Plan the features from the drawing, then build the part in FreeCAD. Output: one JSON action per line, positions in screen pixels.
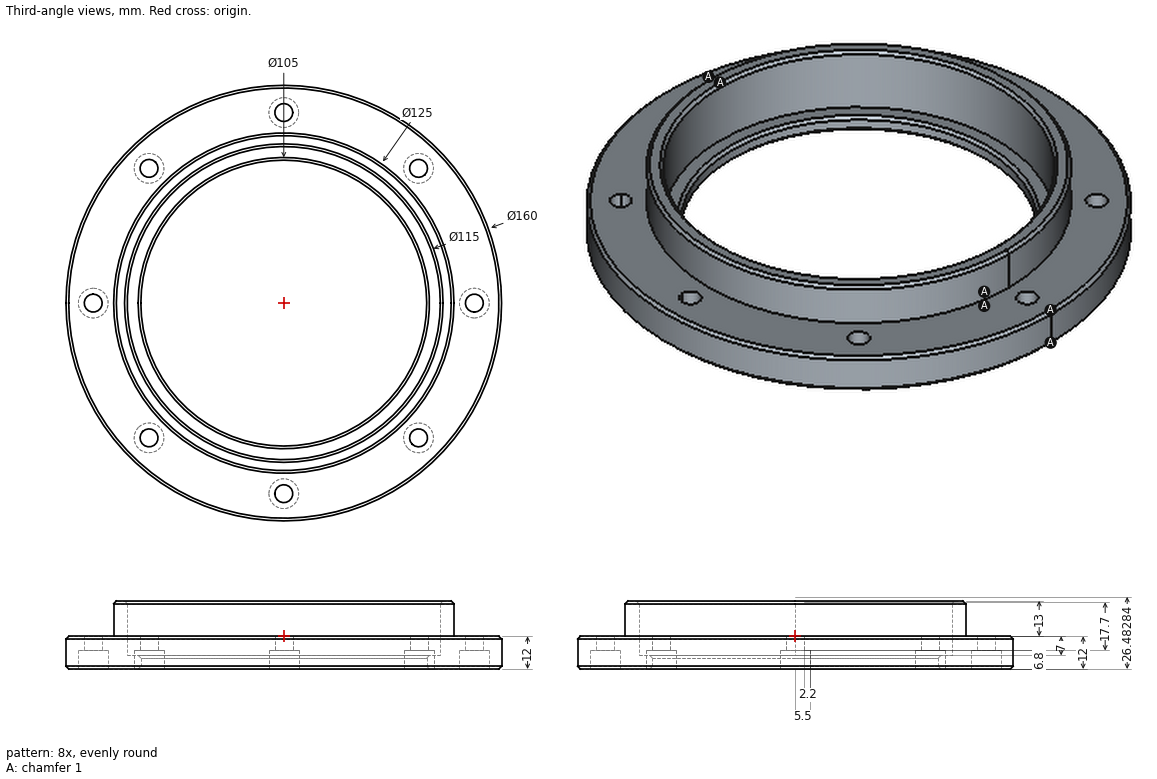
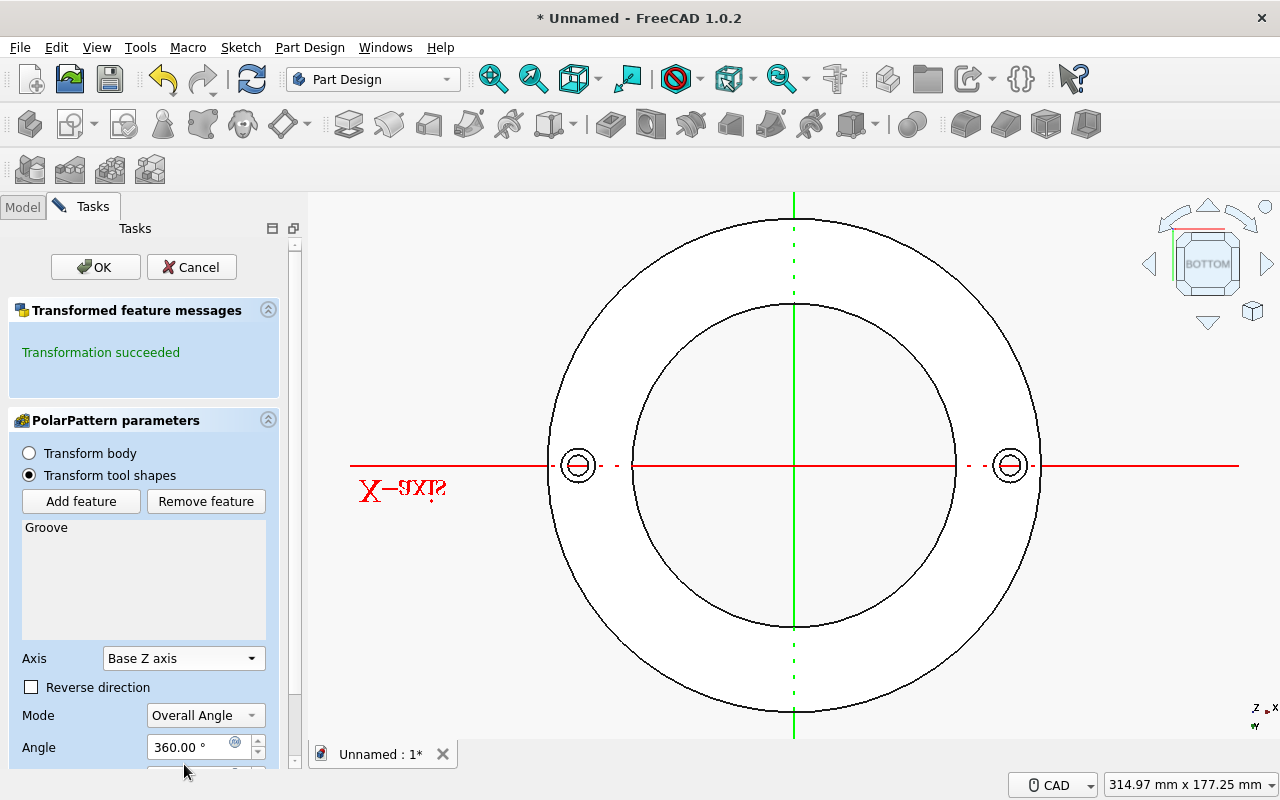
{"action": "scroll", "coordinate": [295, 503], "scroll_direction": "down", "scroll_amount": 2}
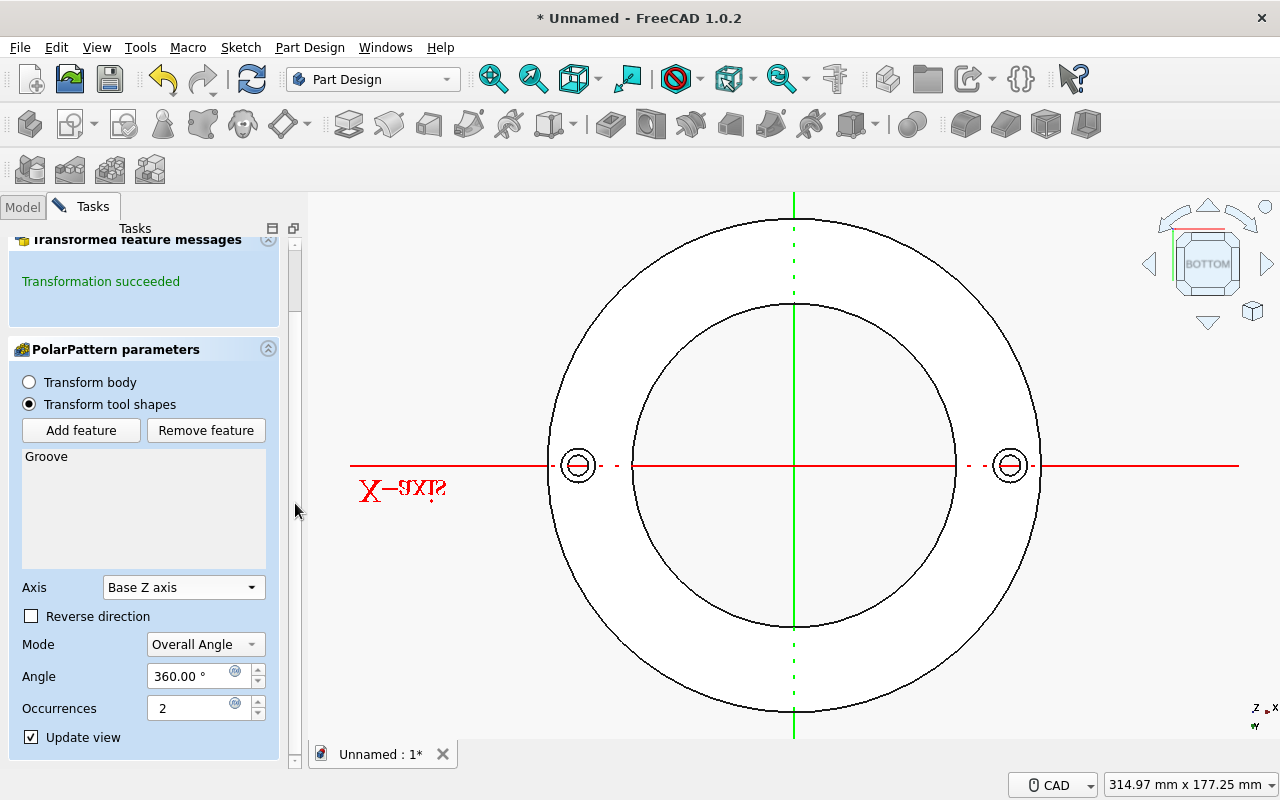
{"action": "triple_click", "coordinate": [198, 708]}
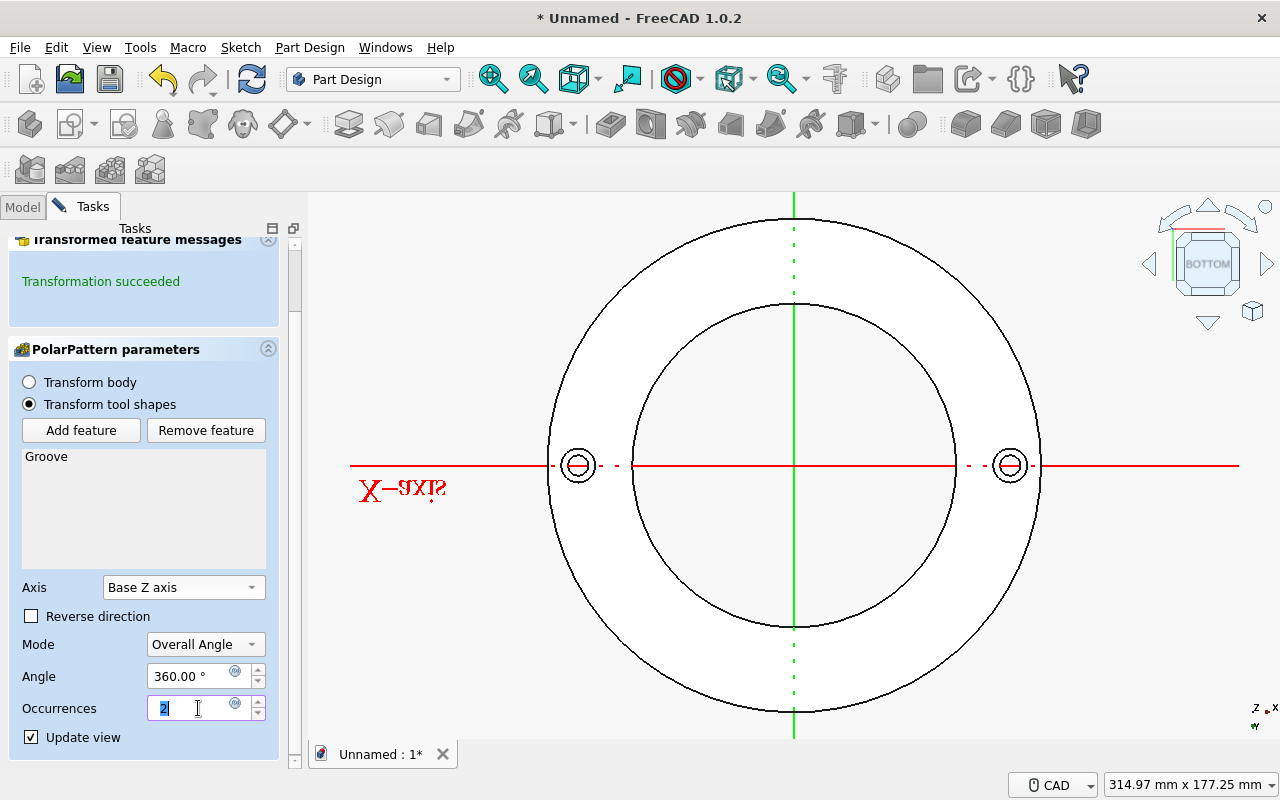
{"action": "type", "text": "8"}
{"action": "key", "text": "Tab"}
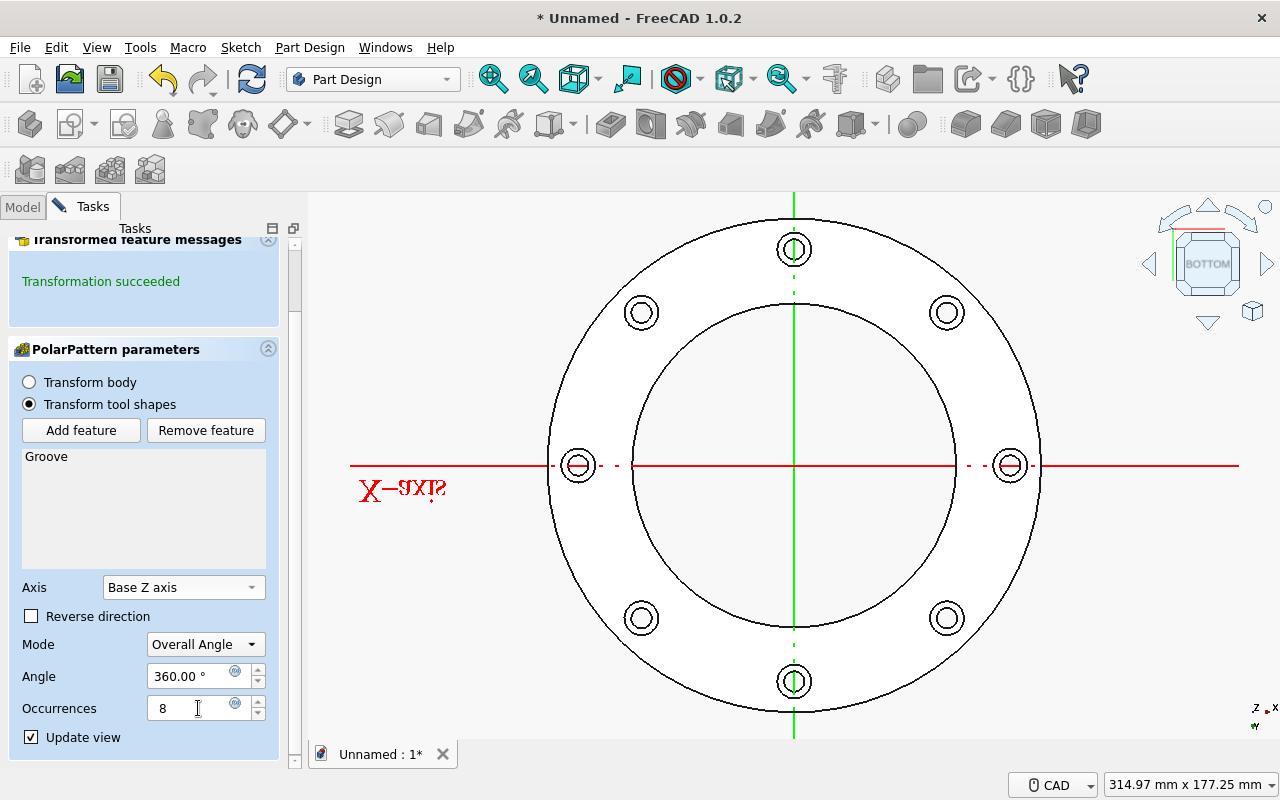
{"action": "scroll", "coordinate": [295, 503], "scroll_direction": "up", "scroll_amount": 2}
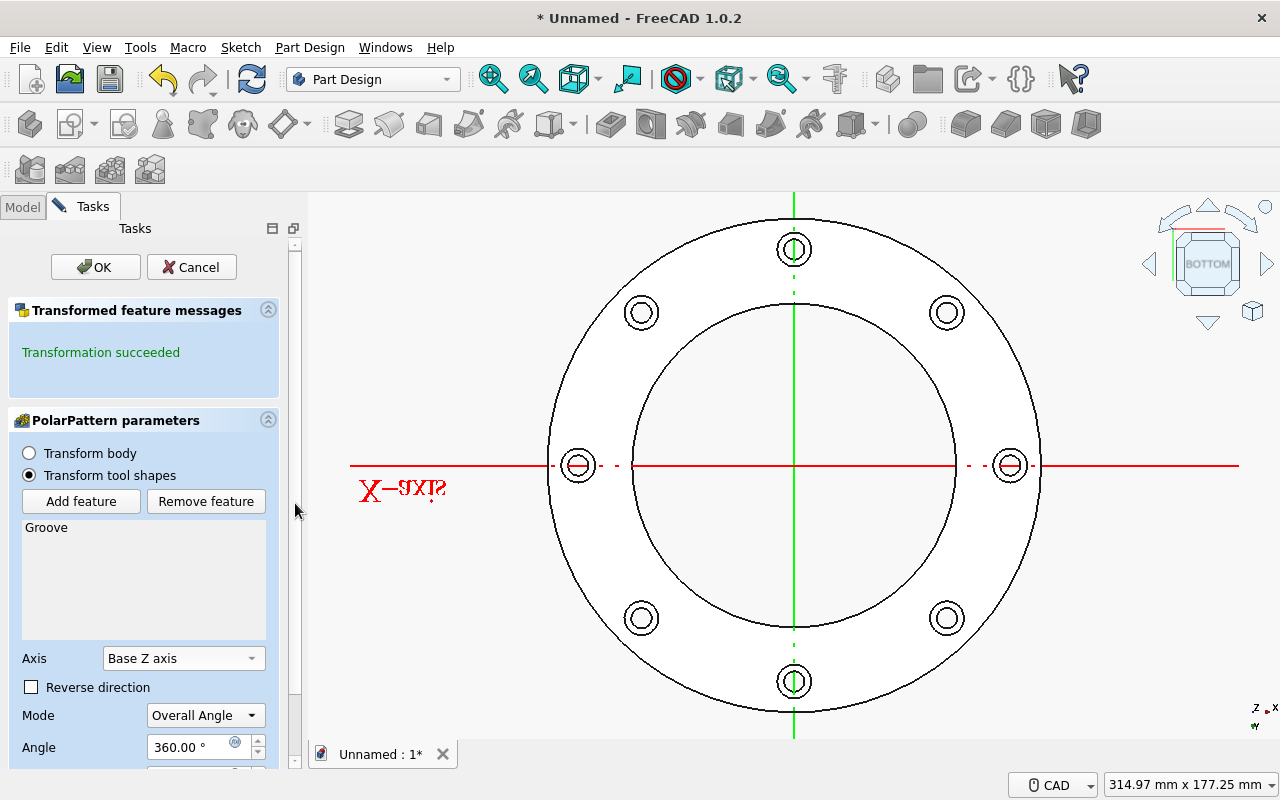
{"action": "left_click", "coordinate": [96, 267]}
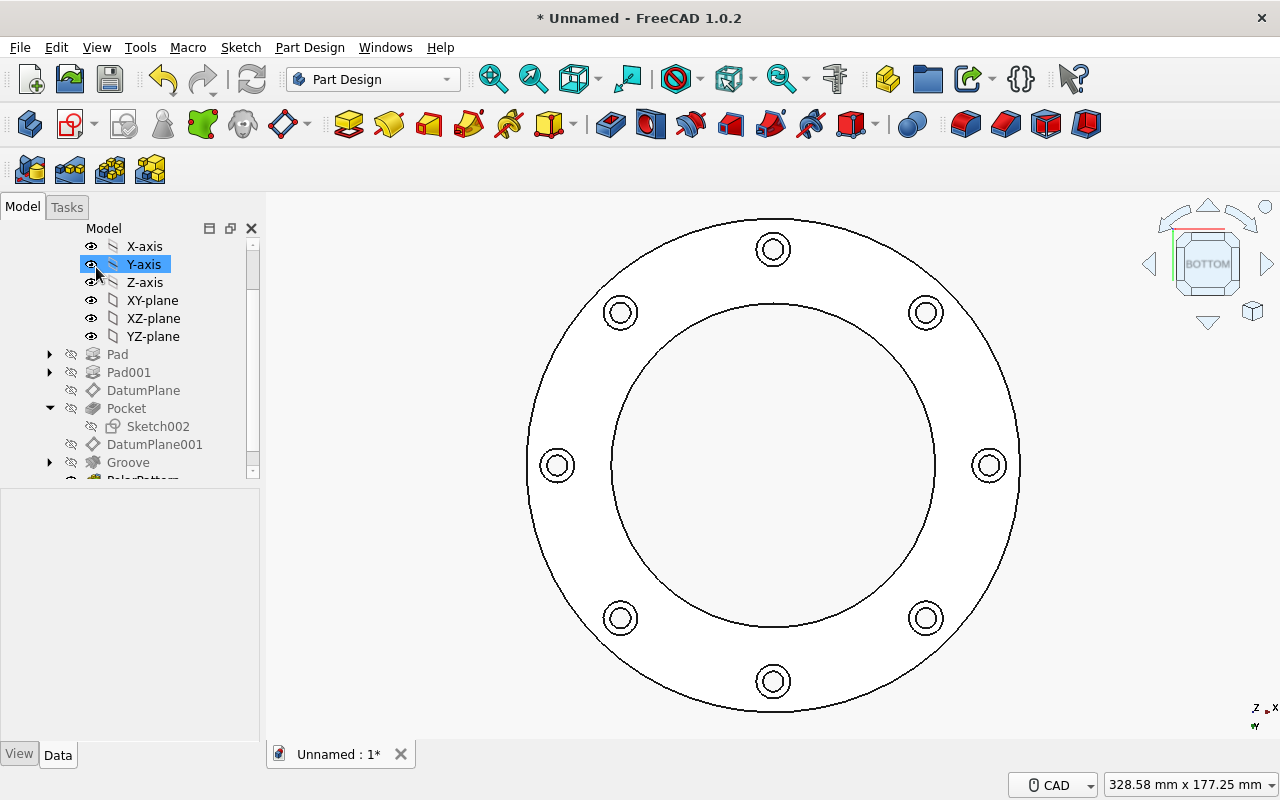
{"action": "left_click", "coordinate": [526, 465]}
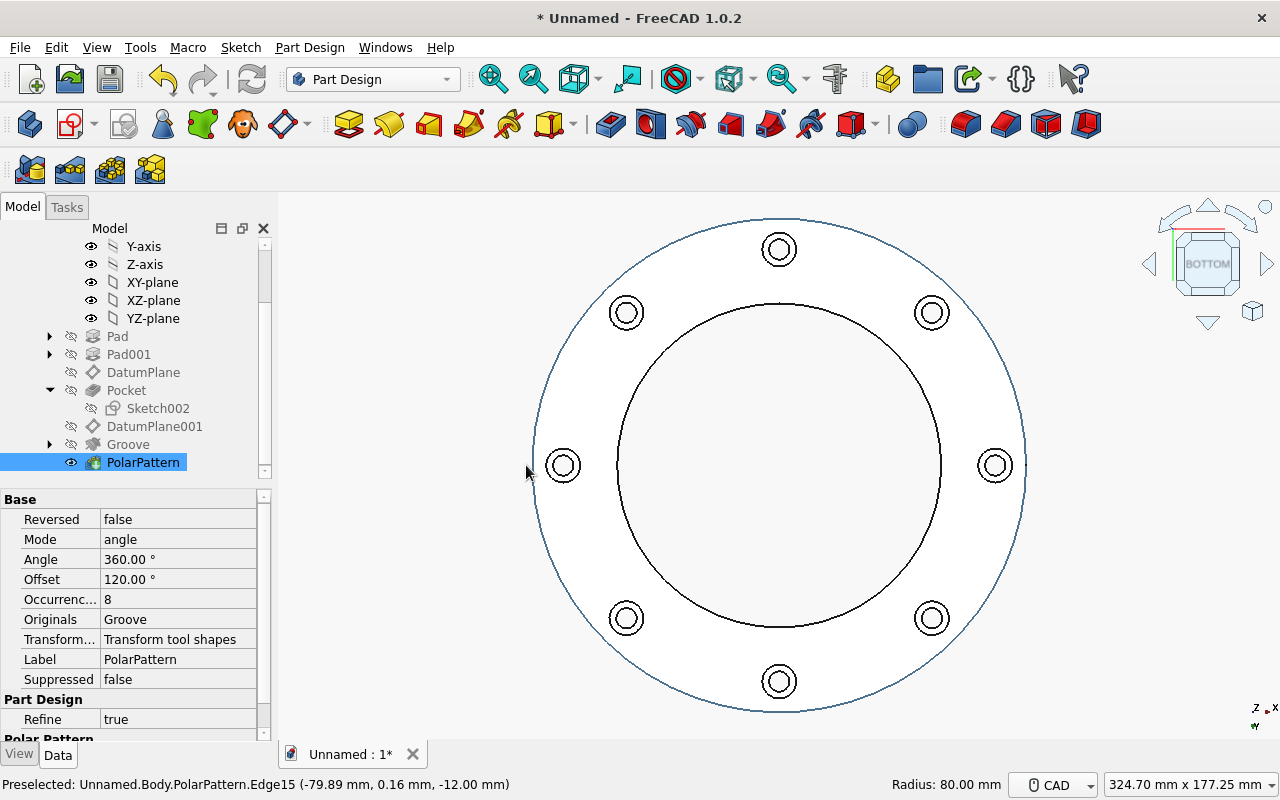
{"action": "left_click", "coordinate": [648, 369], "text": "ctrl"}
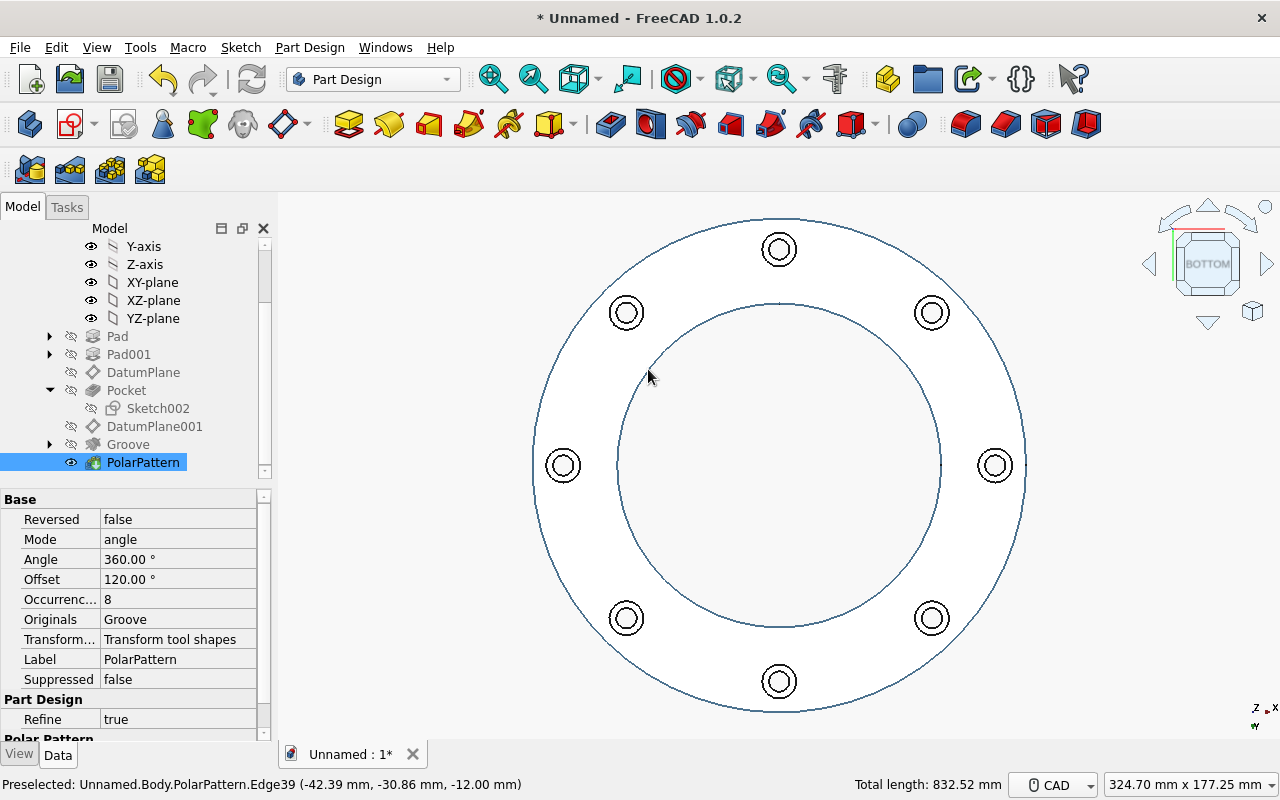
{"action": "key", "text": "0"}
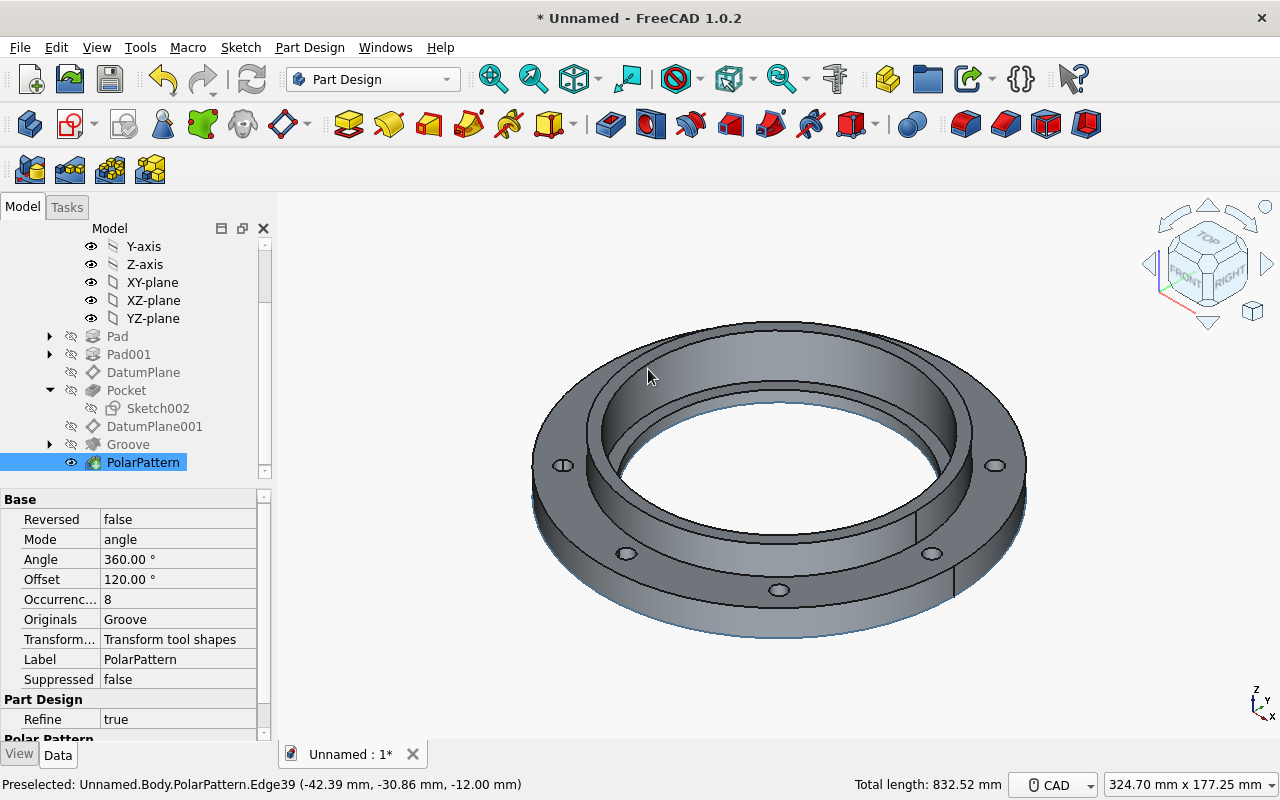
{"action": "left_click", "coordinate": [559, 529], "text": "ctrl"}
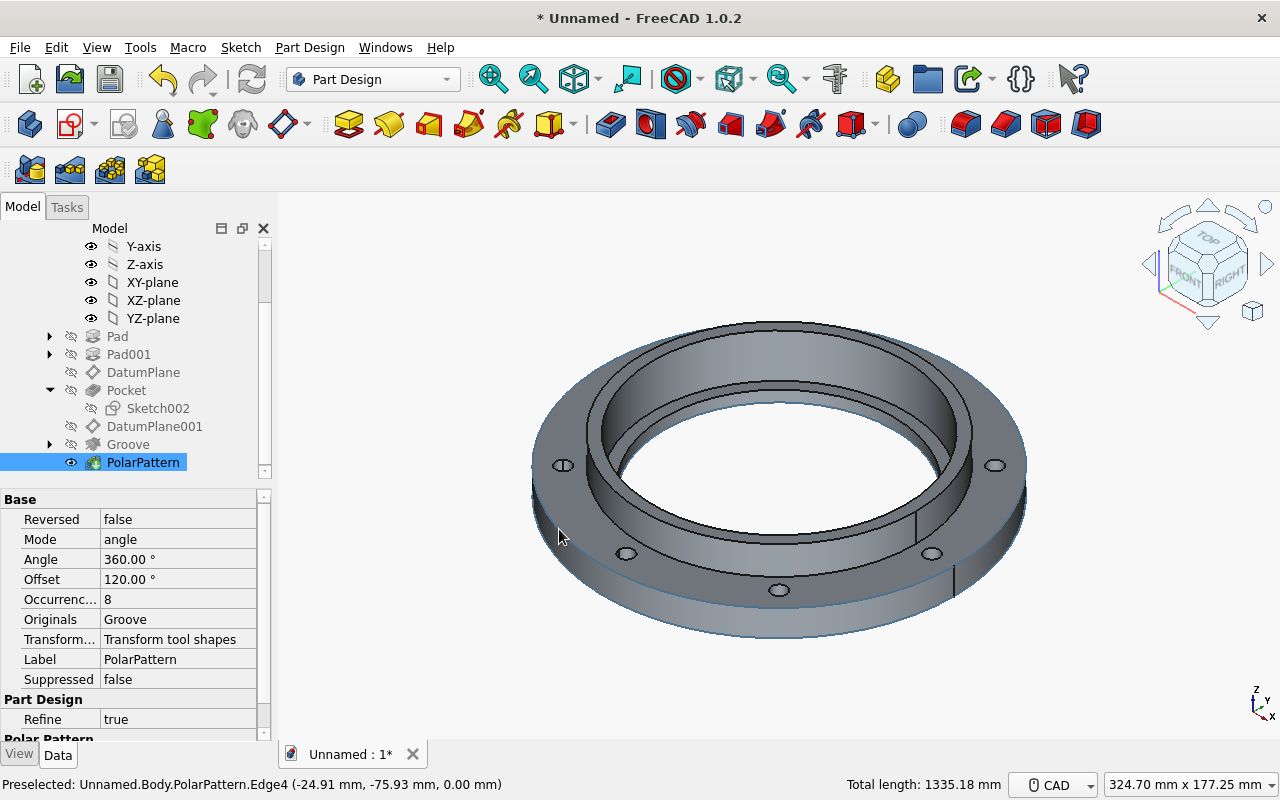
{"action": "left_click", "coordinate": [665, 416], "text": "ctrl"}